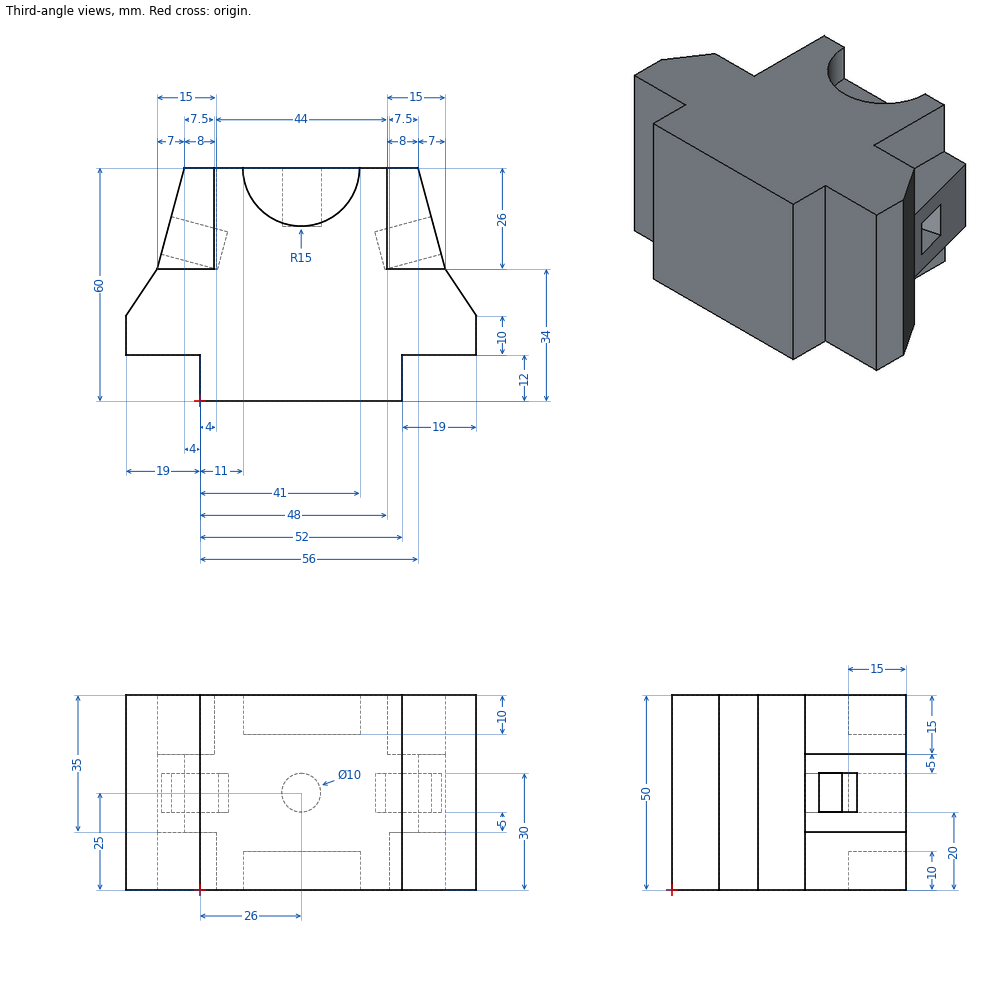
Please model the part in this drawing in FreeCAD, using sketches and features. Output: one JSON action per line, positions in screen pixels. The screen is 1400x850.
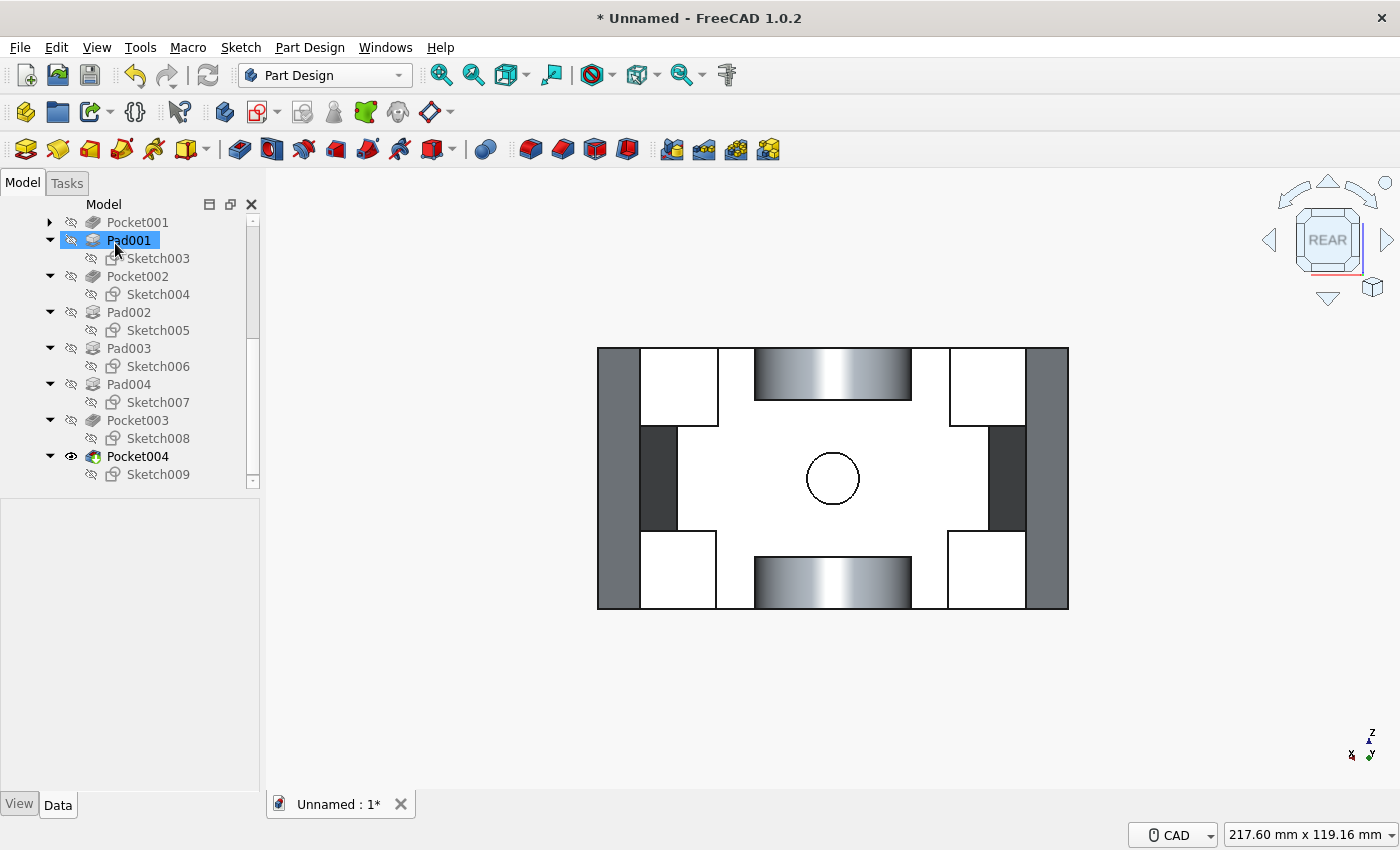
{"action": "left_click", "coordinate": [442, 76]}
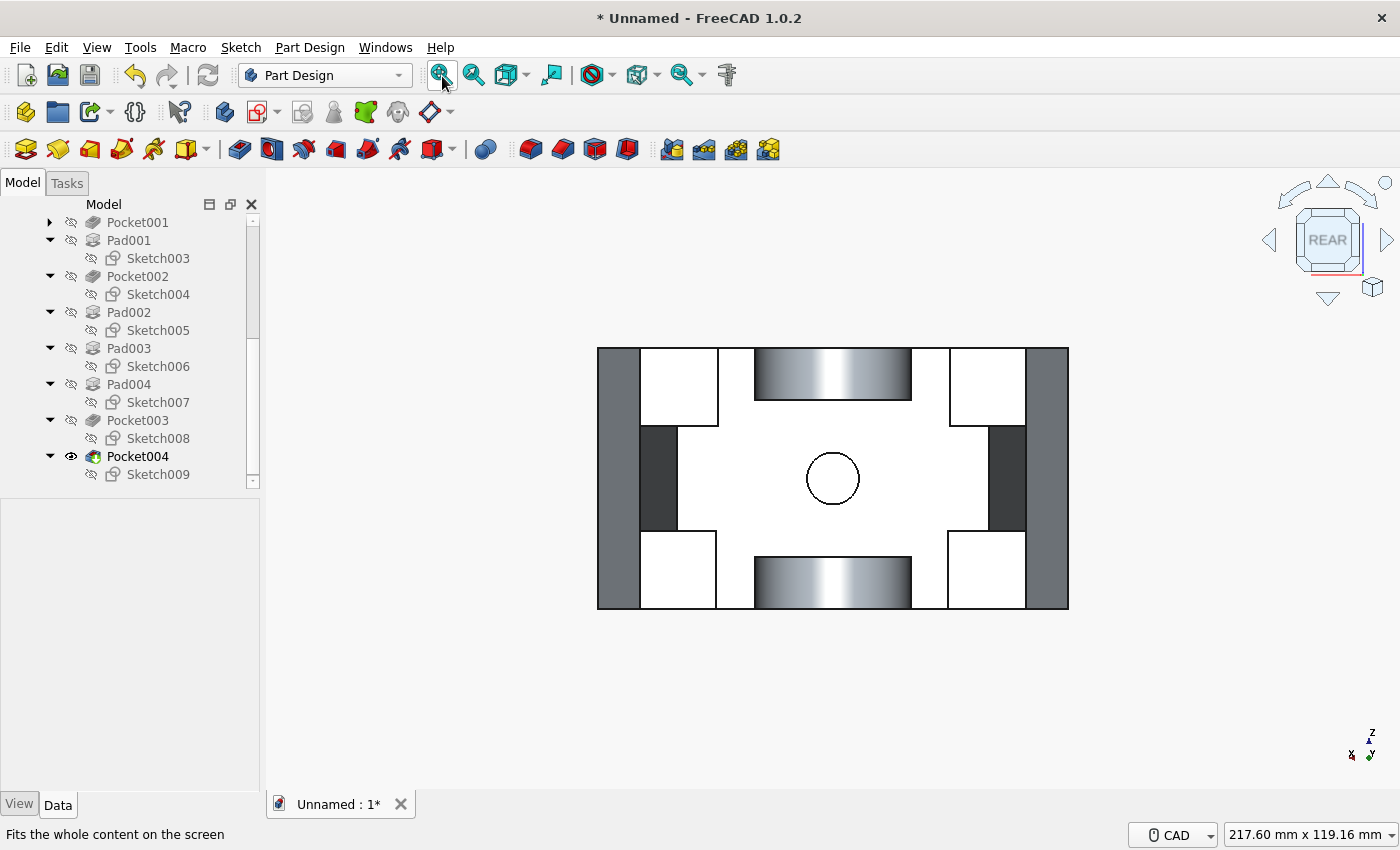
{"action": "left_click", "coordinate": [1008, 477]}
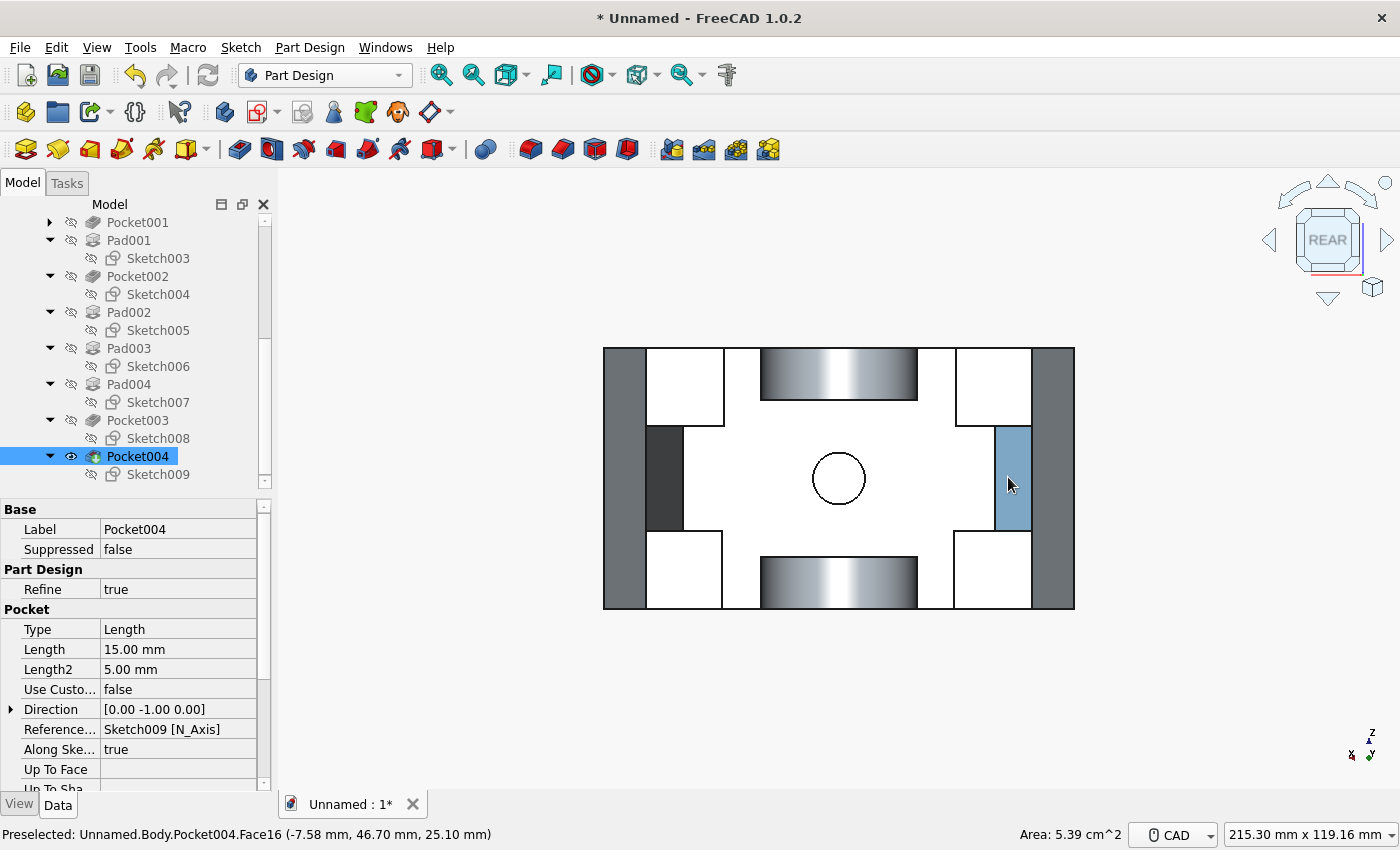
{"action": "left_click", "coordinate": [258, 112]}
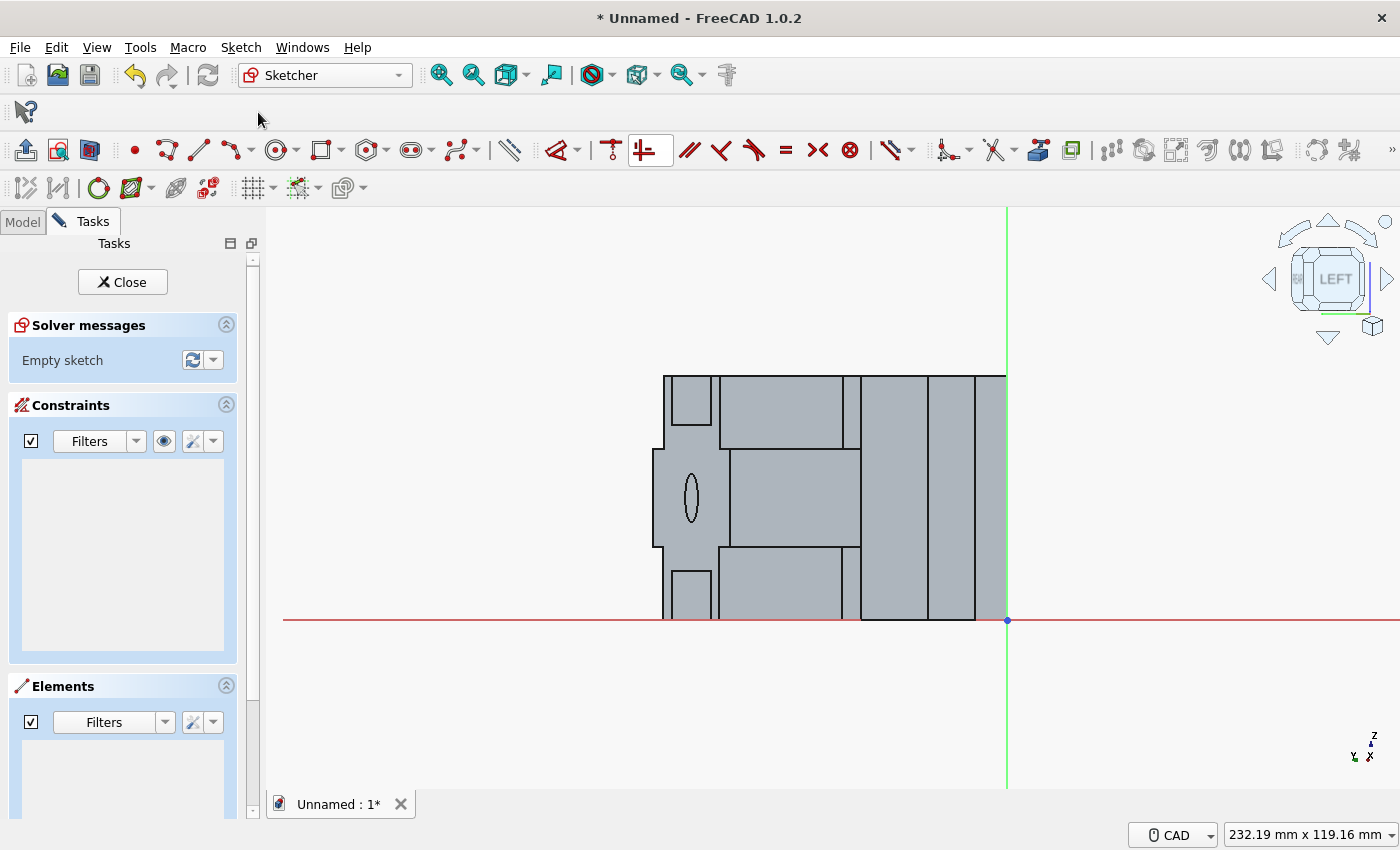
{"action": "scroll", "coordinate": [826, 498], "scroll_direction": "up", "scroll_amount": 10}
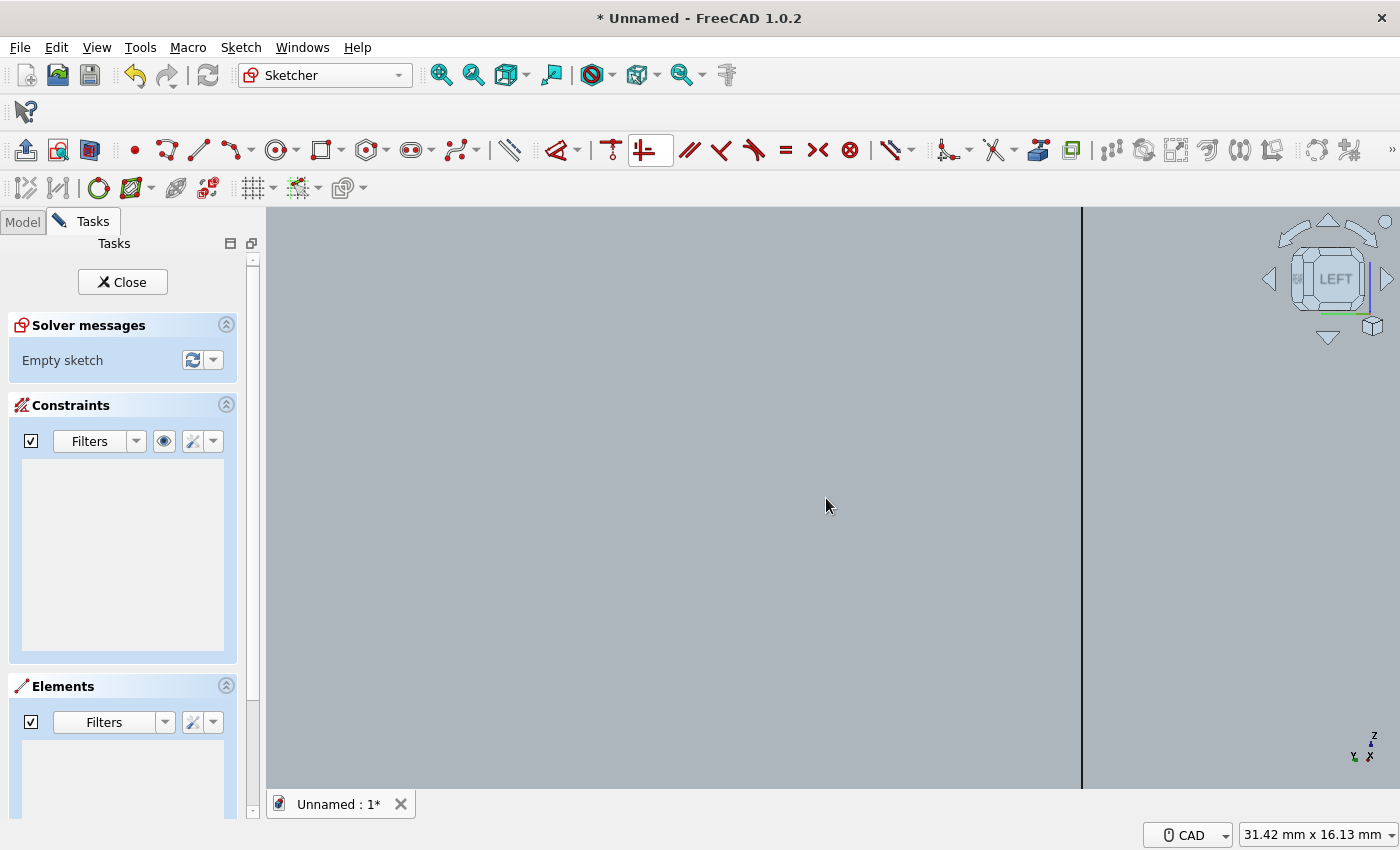
{"action": "left_click", "coordinate": [322, 150]}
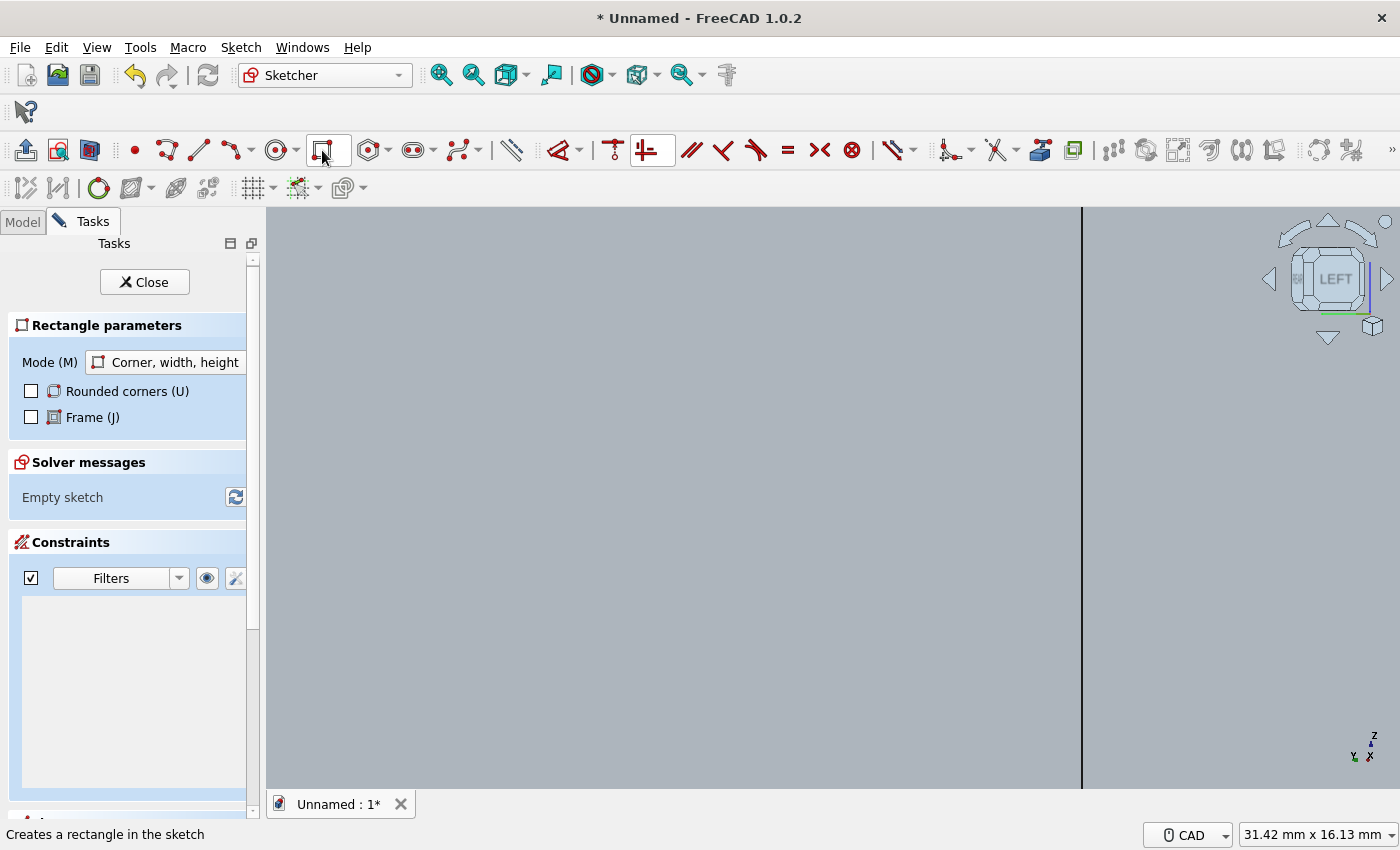
{"action": "left_click", "coordinate": [580, 314]}
{"action": "left_click", "coordinate": [941, 675]}
{"action": "key", "text": "Escape"}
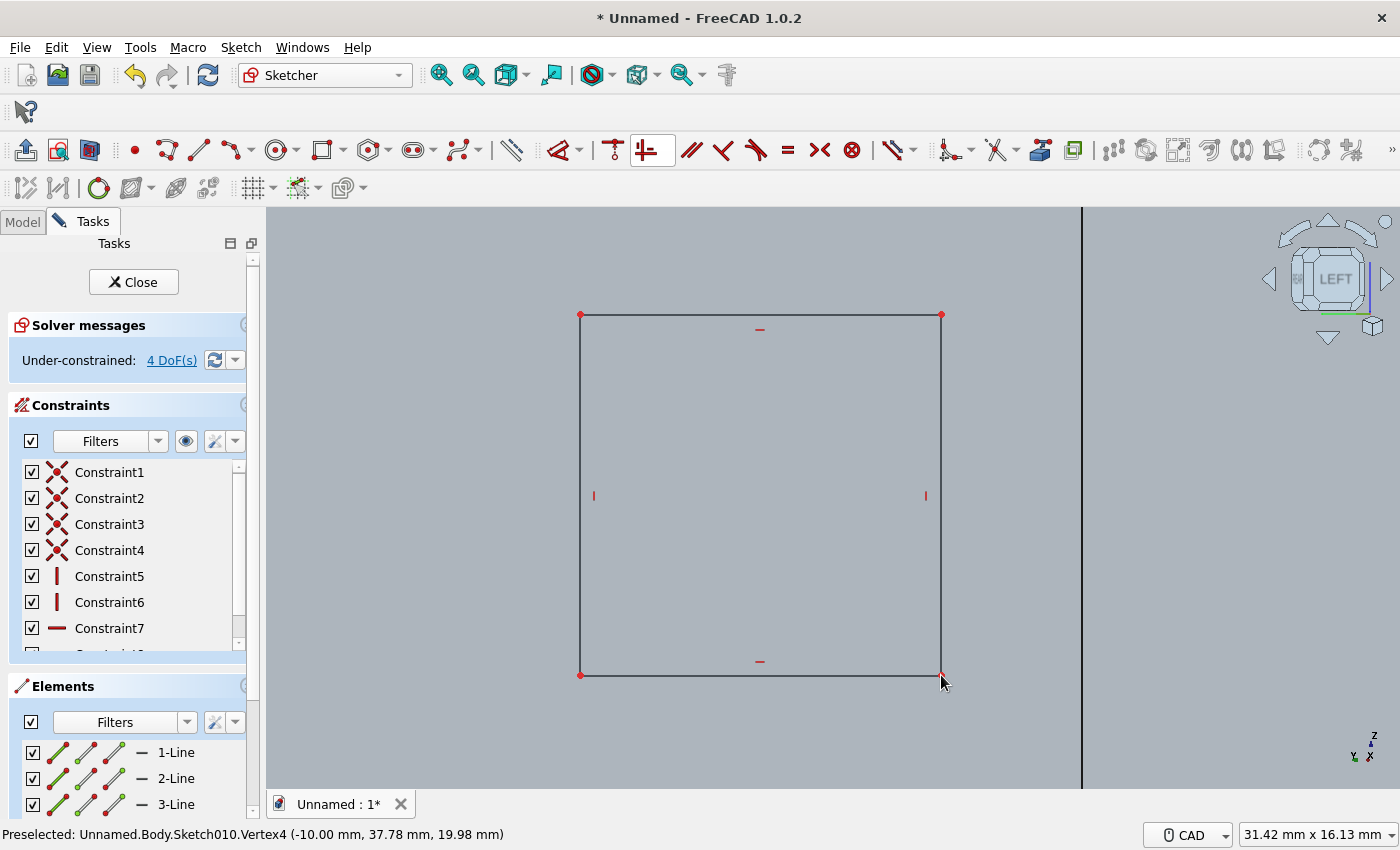
{"action": "left_click", "coordinate": [558, 150]}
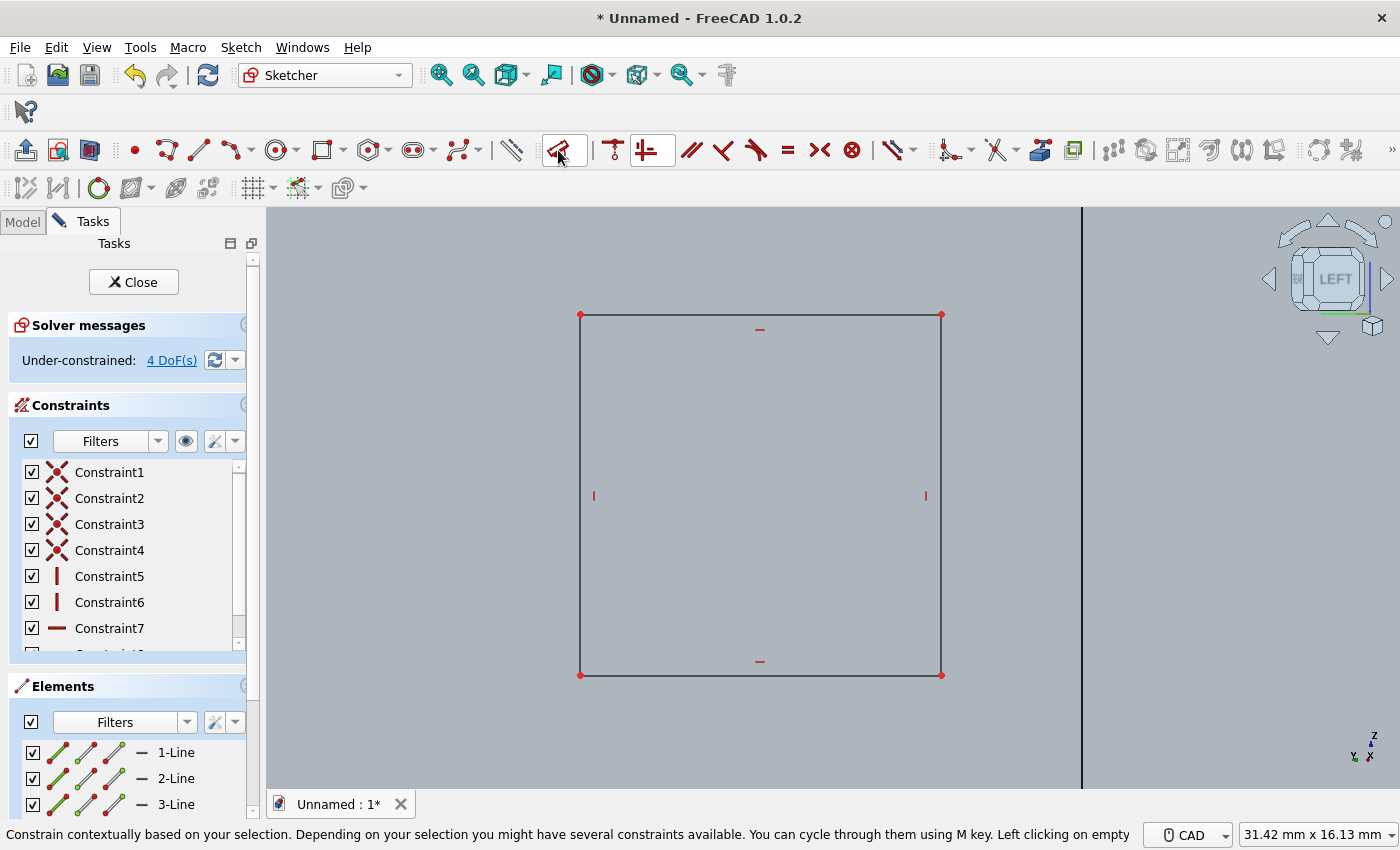
{"action": "left_click", "coordinate": [580, 423]}
{"action": "left_click", "coordinate": [546, 495]}